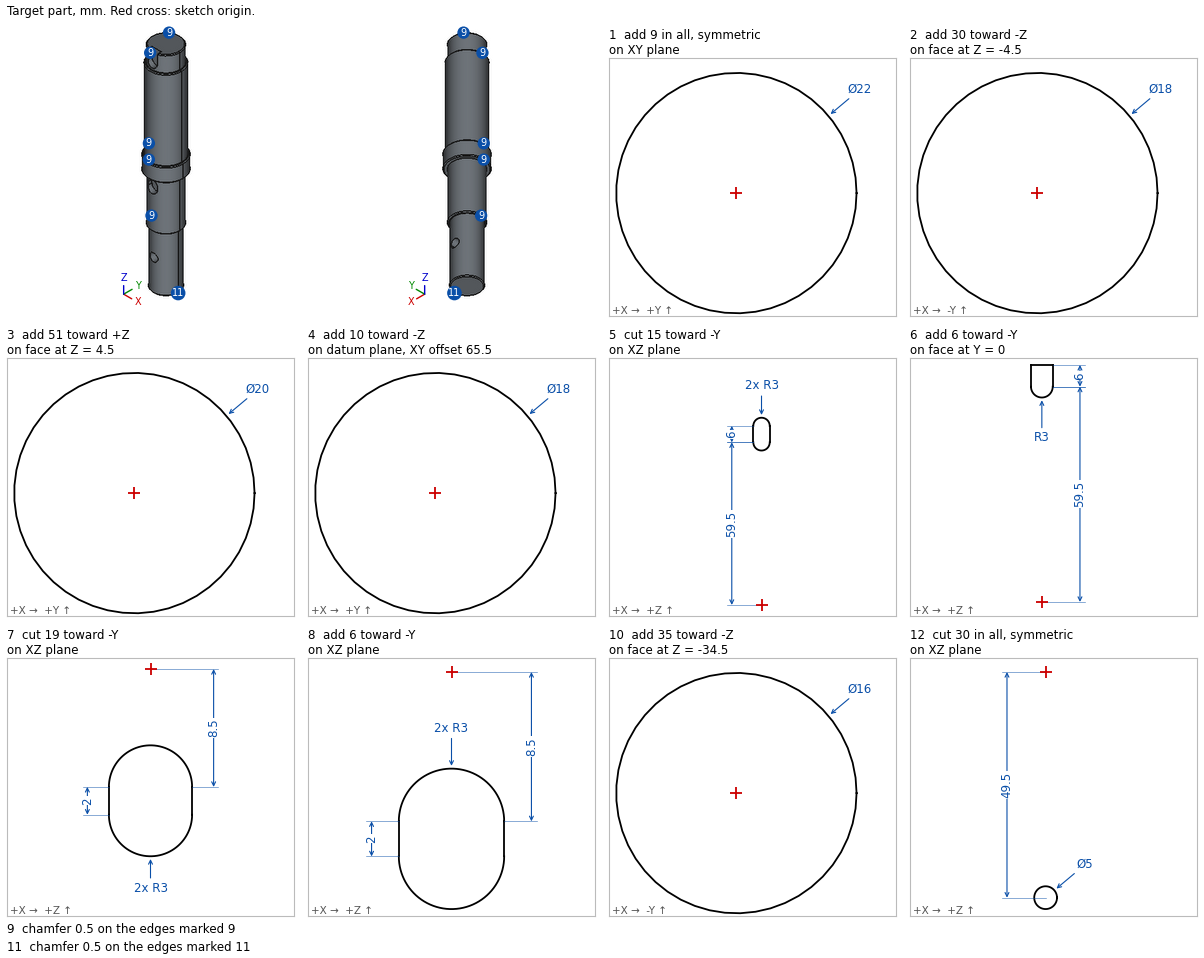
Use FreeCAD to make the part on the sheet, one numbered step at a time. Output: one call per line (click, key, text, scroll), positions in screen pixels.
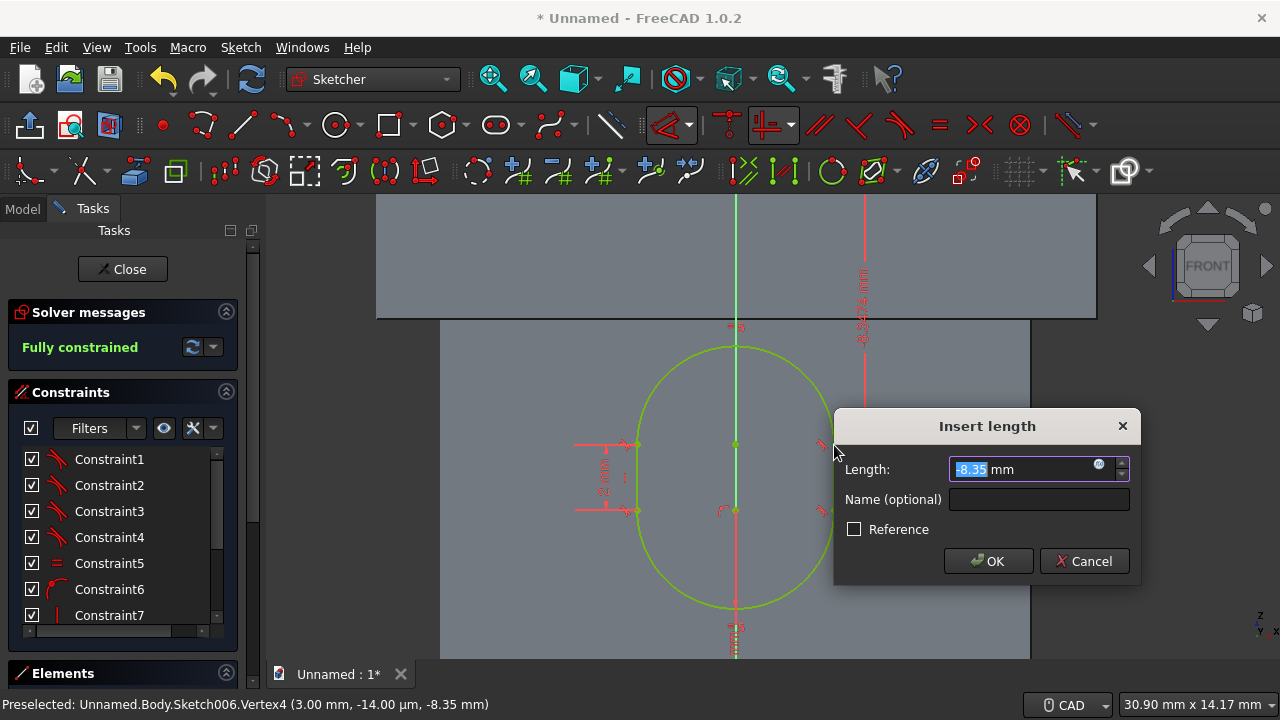
text(-8.5)
key(Return)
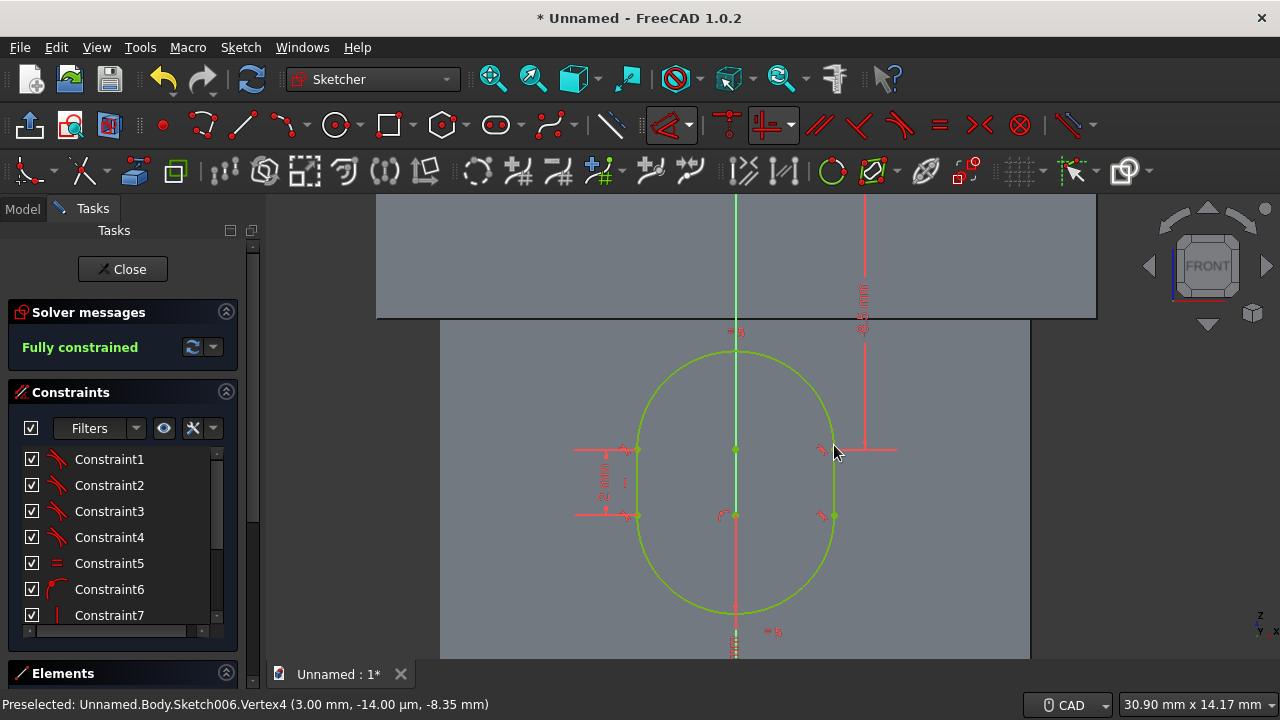
click(123, 269)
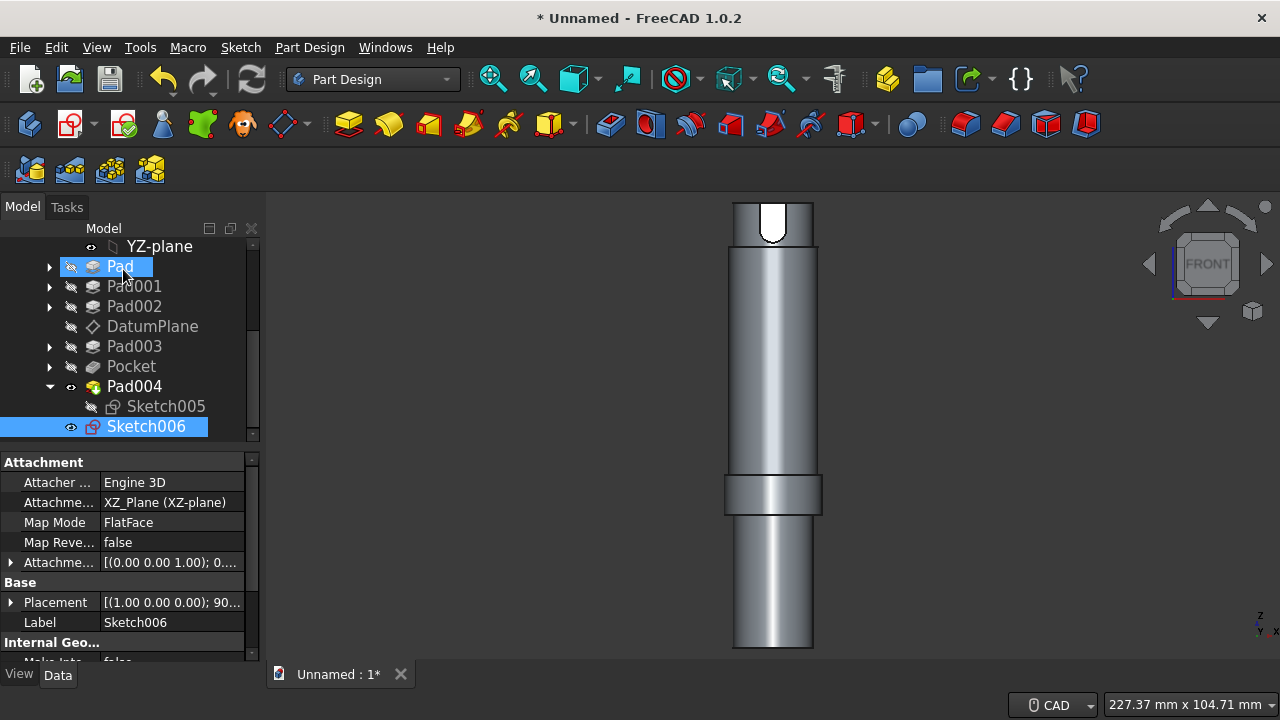
click(612, 124)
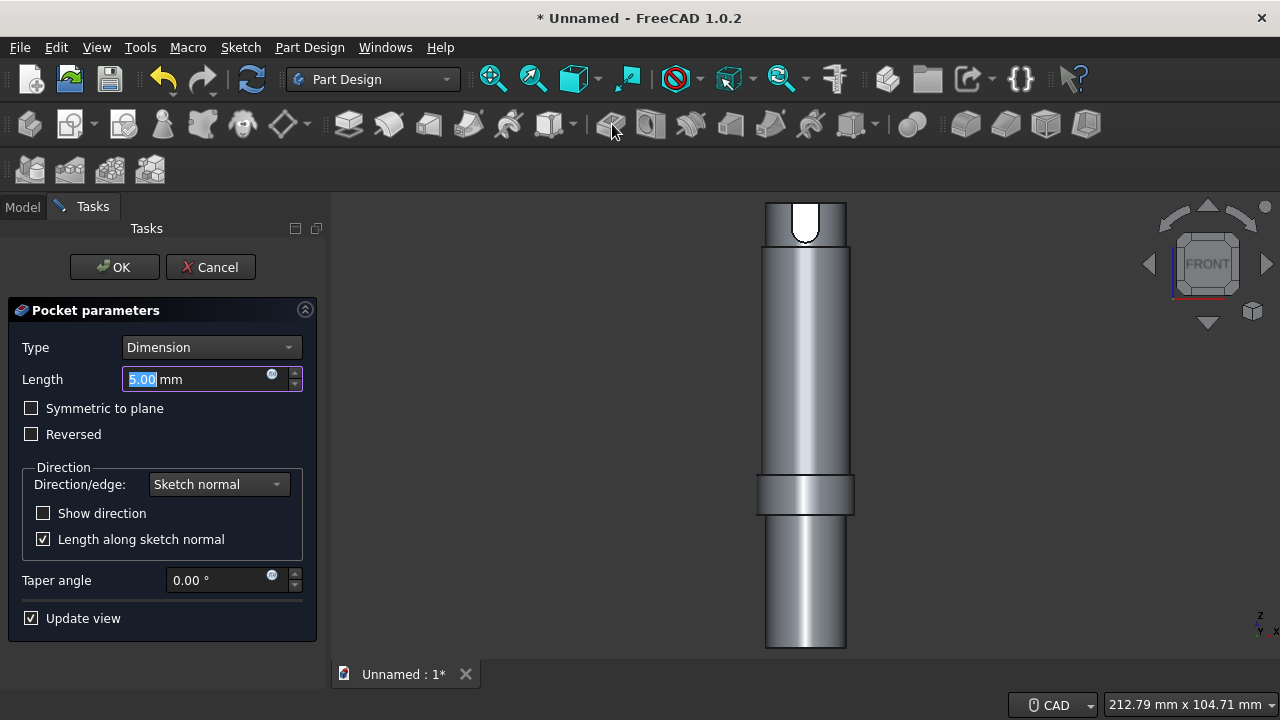
text(19)
key(Tab)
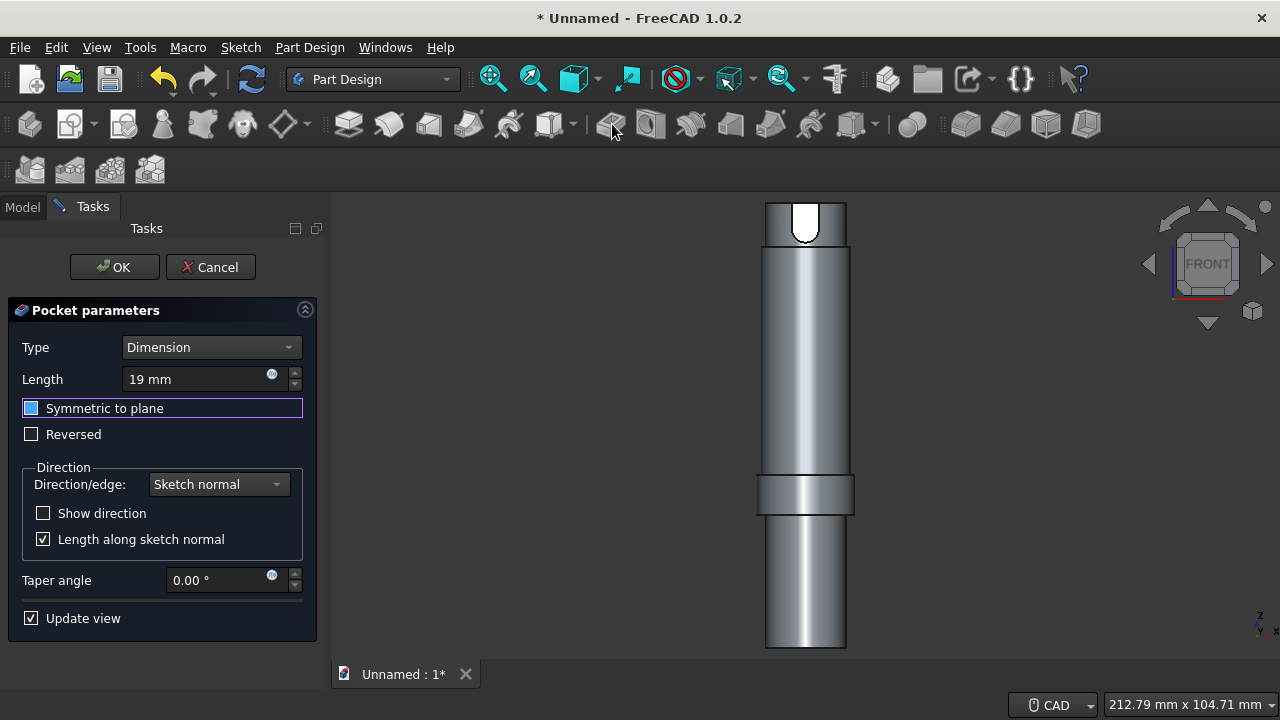
click(30, 434)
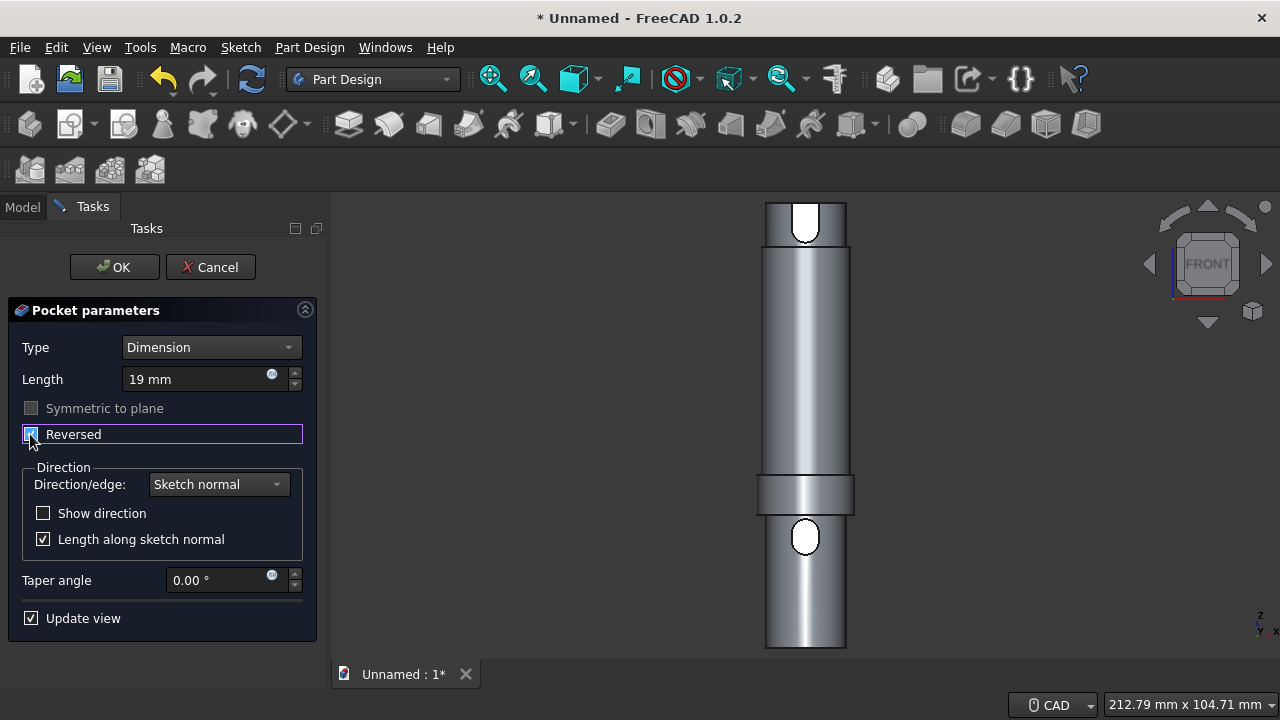
click(115, 267)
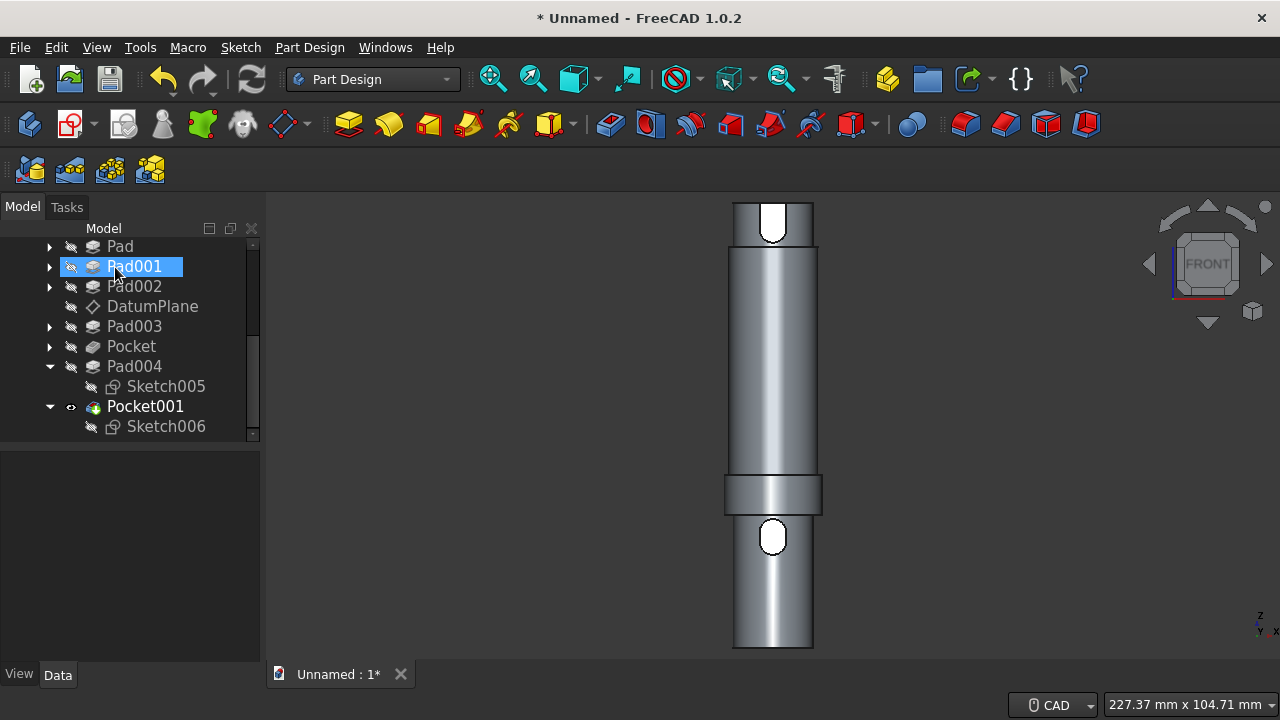
click(70, 124)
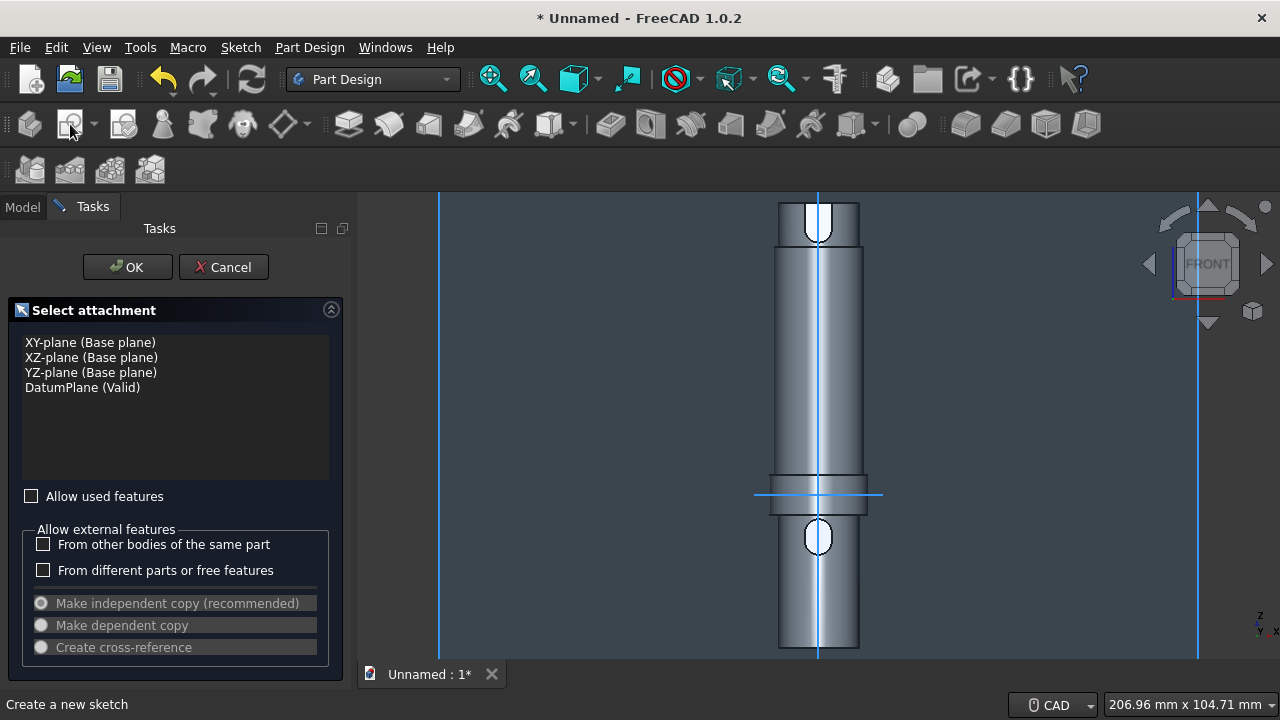
click(82, 358)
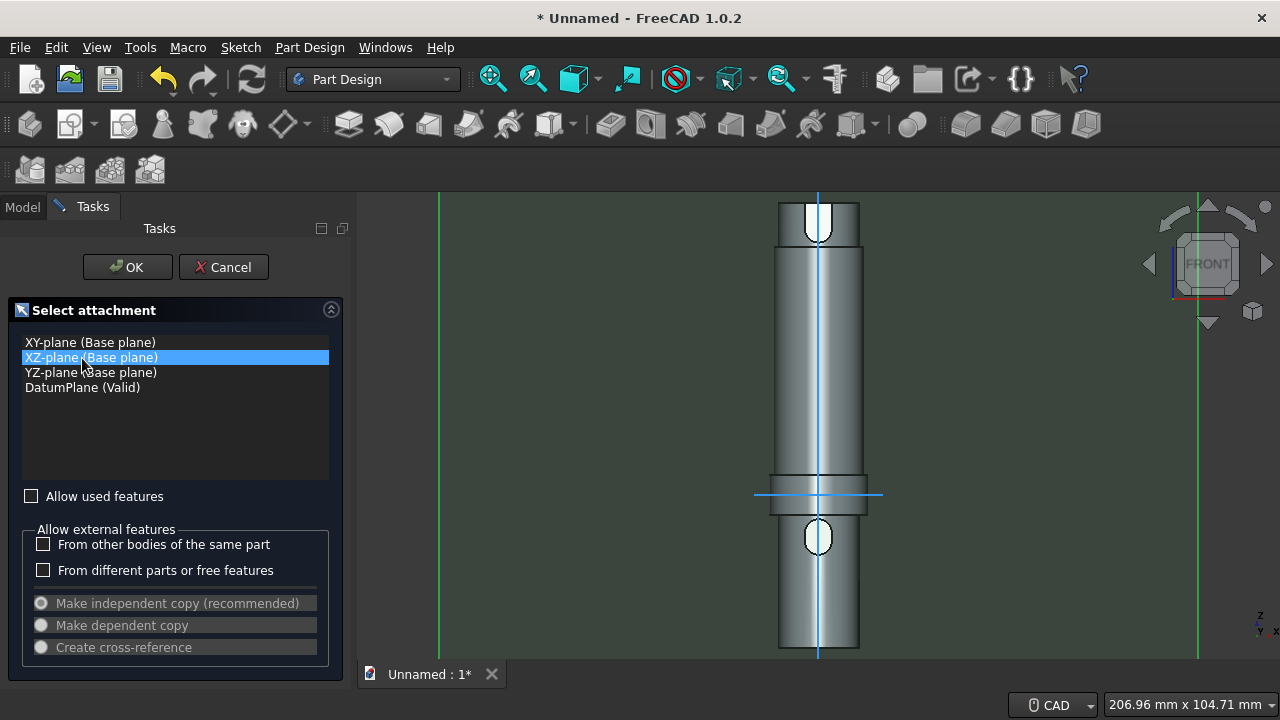
click(128, 267)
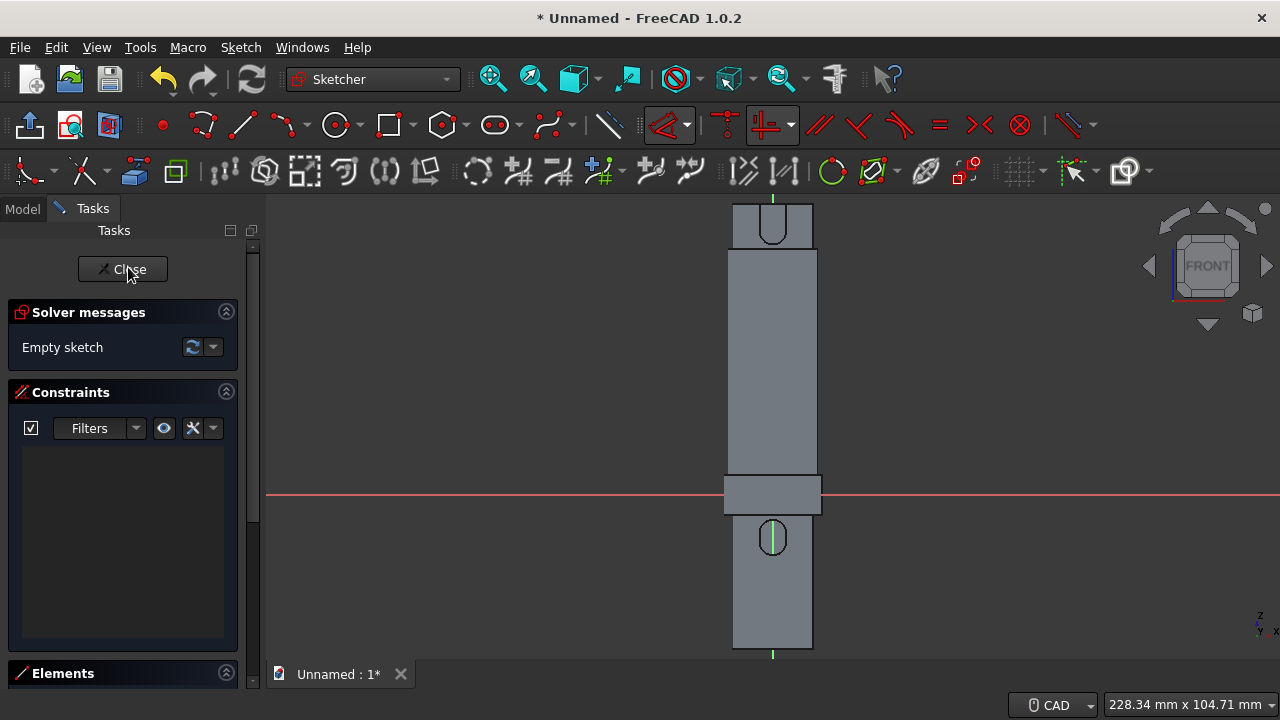
click(110, 126)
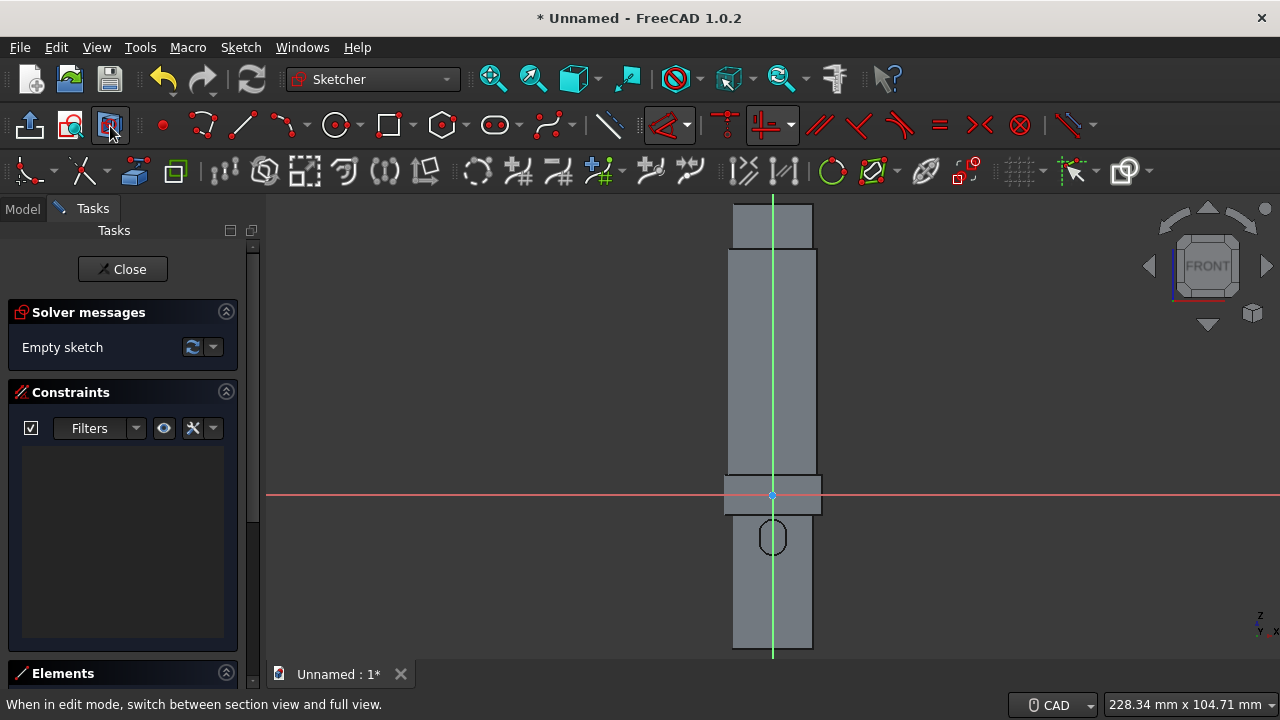
scroll(790, 550, up, 8)